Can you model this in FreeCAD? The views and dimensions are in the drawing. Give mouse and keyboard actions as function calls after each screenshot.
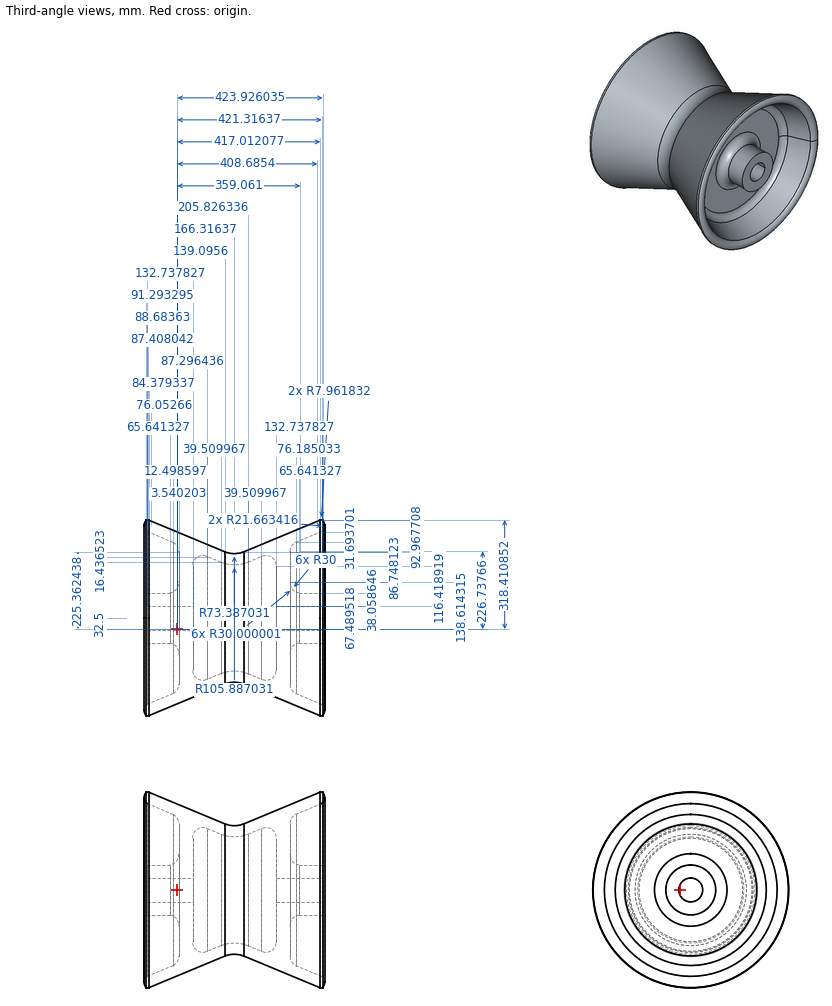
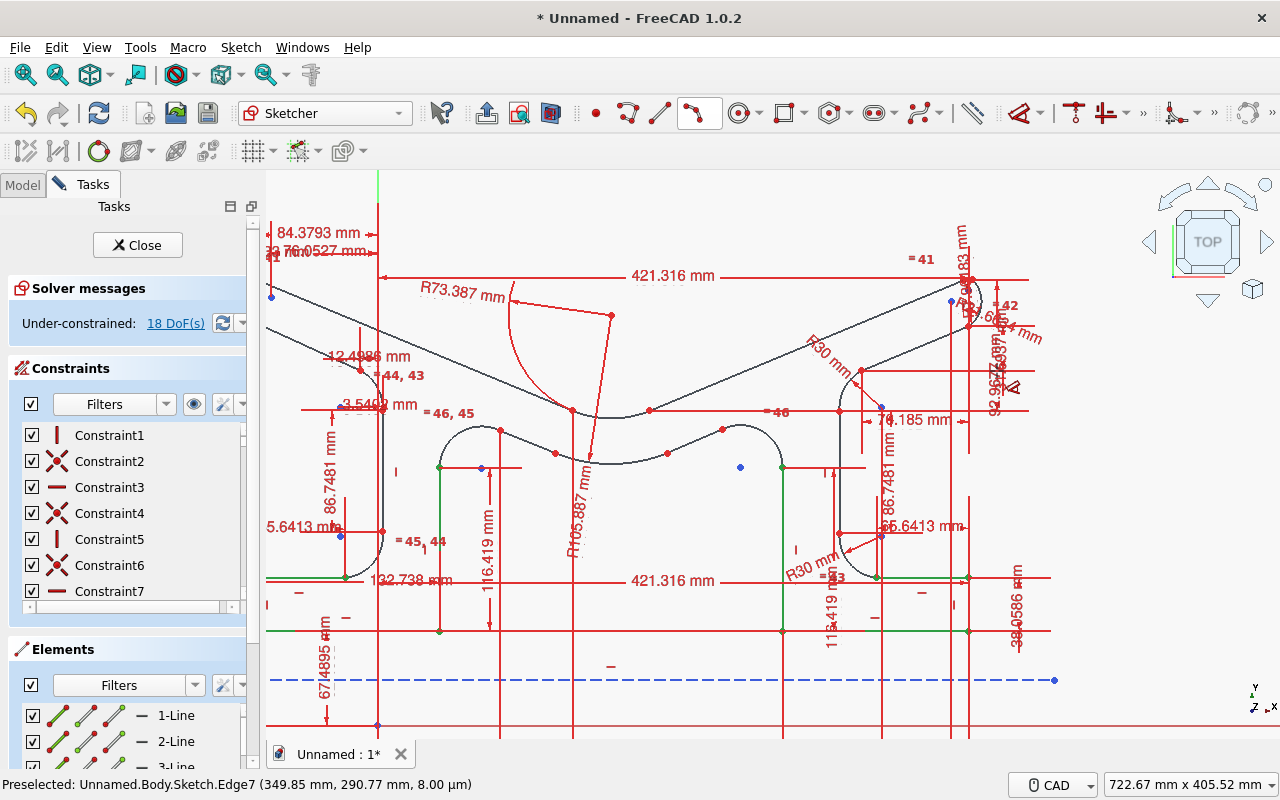
click(479, 372)
click(607, 346)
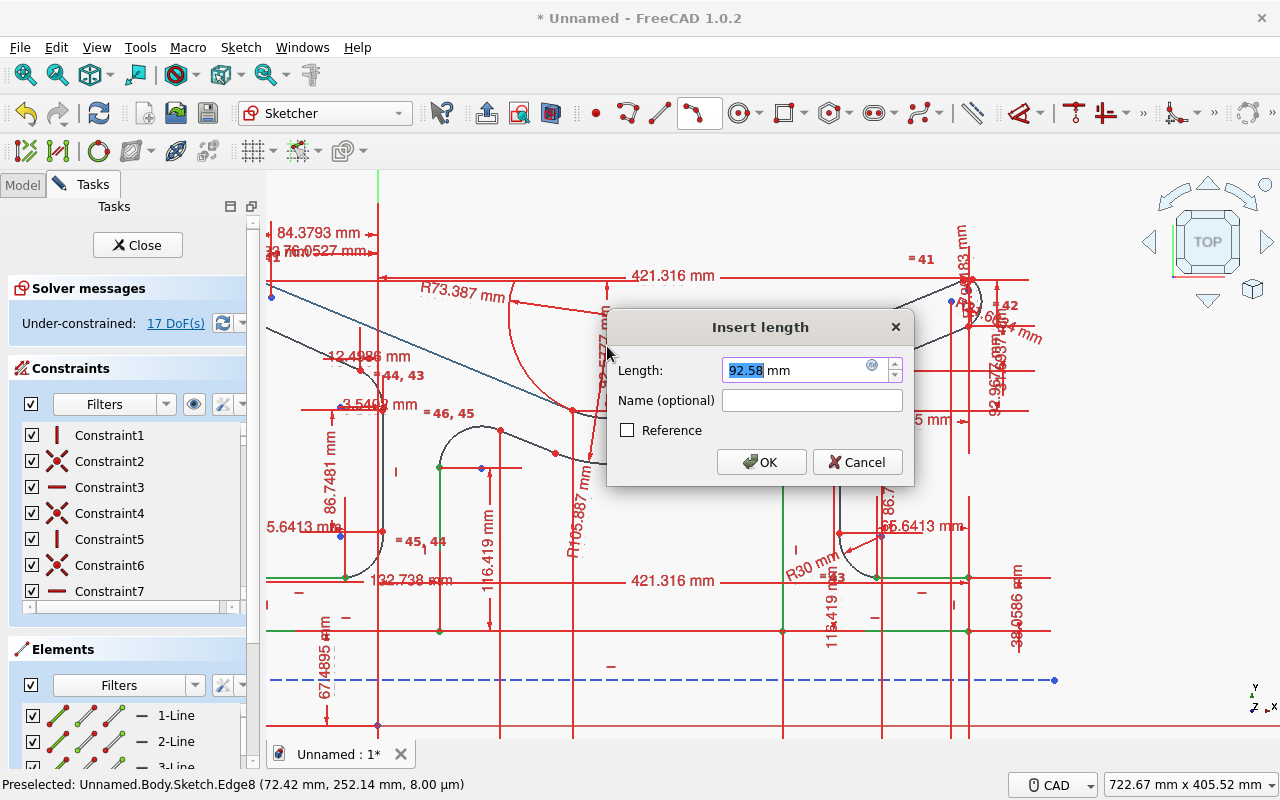
text(92.967708)
key(Return)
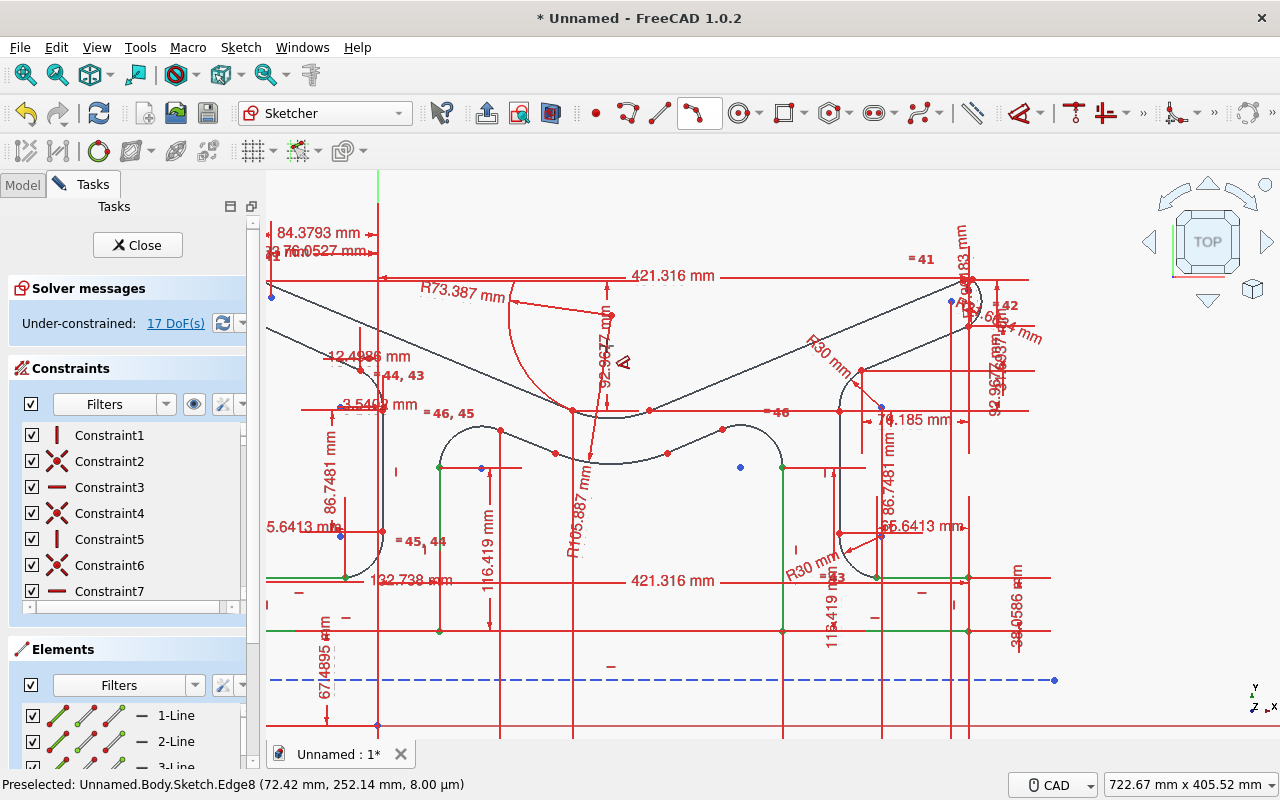
click(328, 356)
click(418, 329)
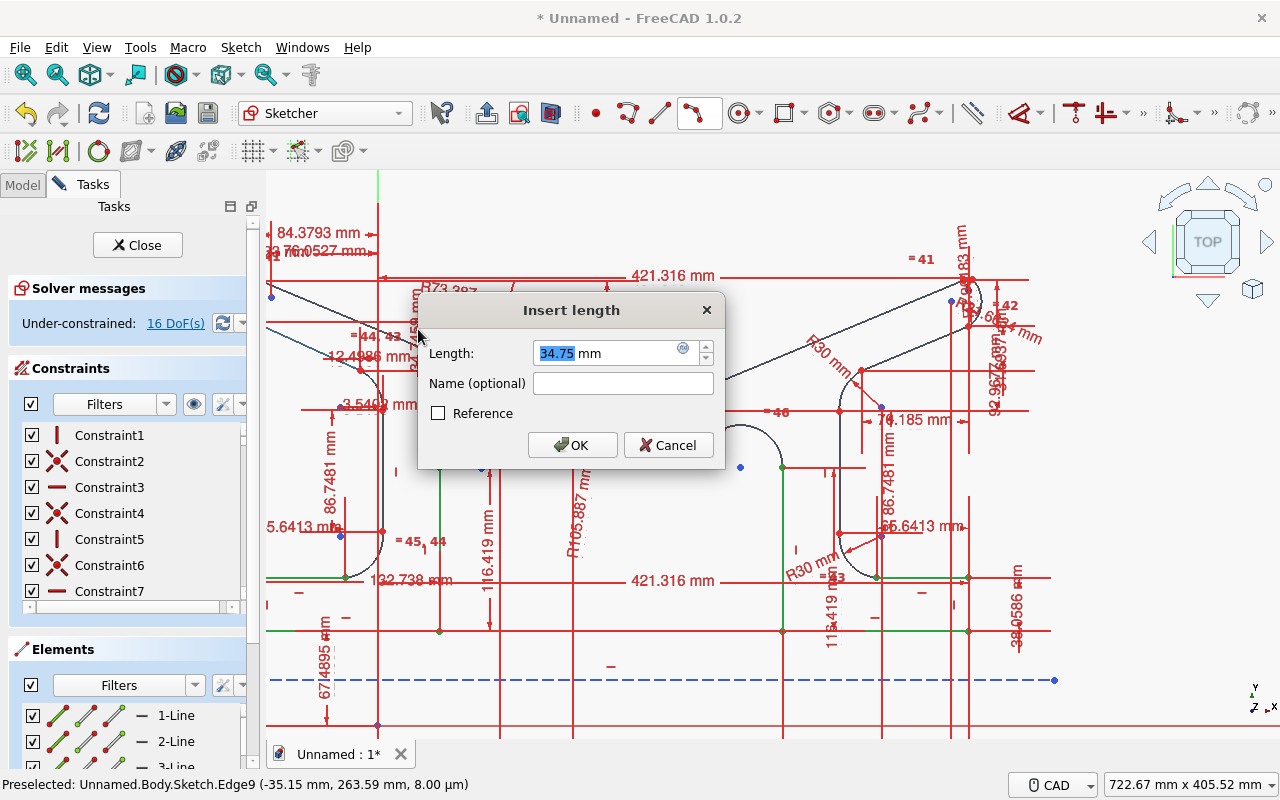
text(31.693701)
key(Return)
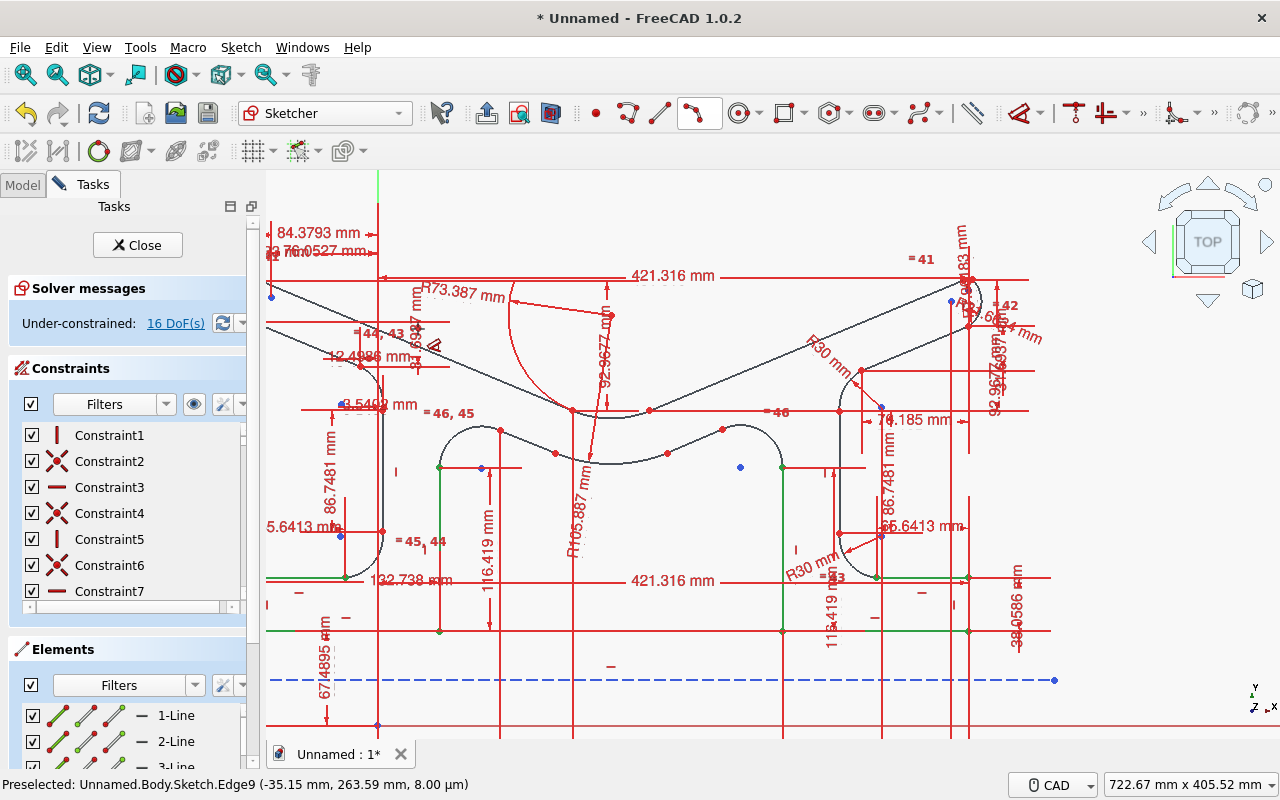
click(517, 437)
click(528, 487)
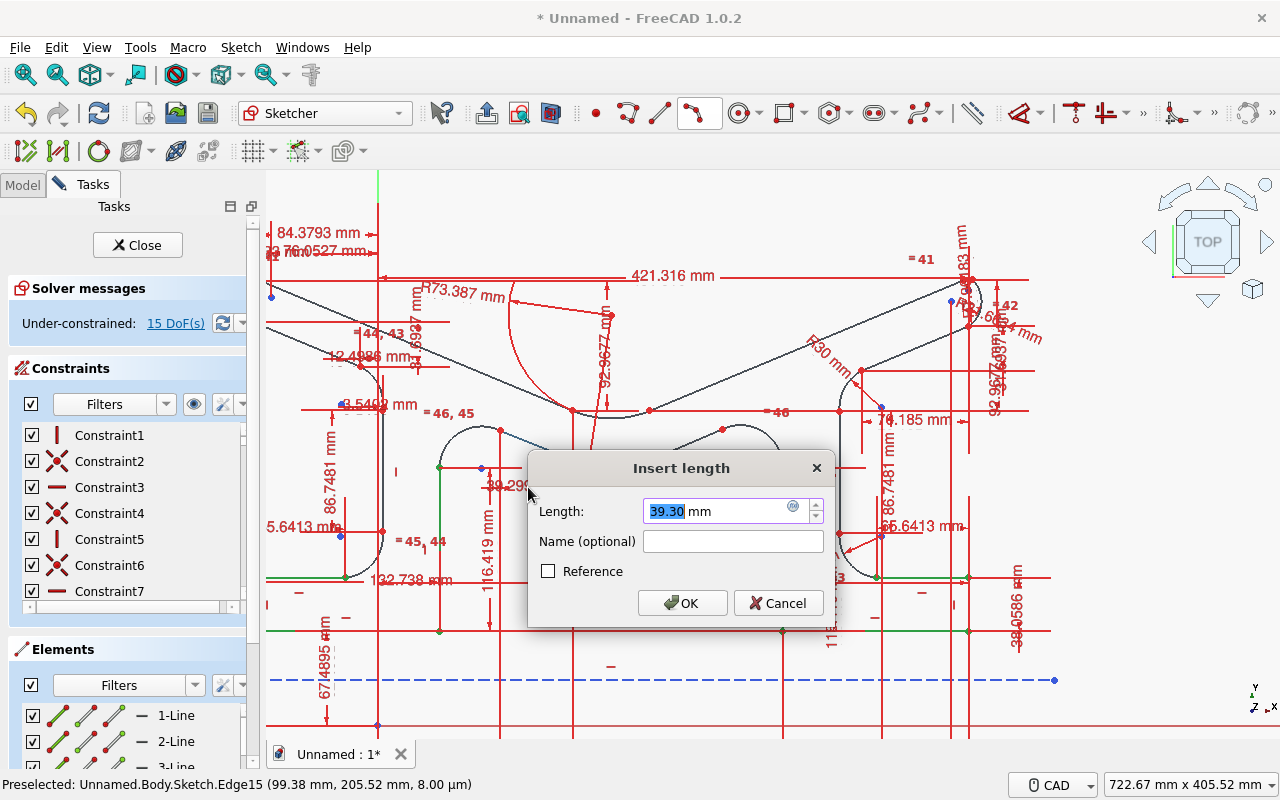
text(39.509967)
key(Return)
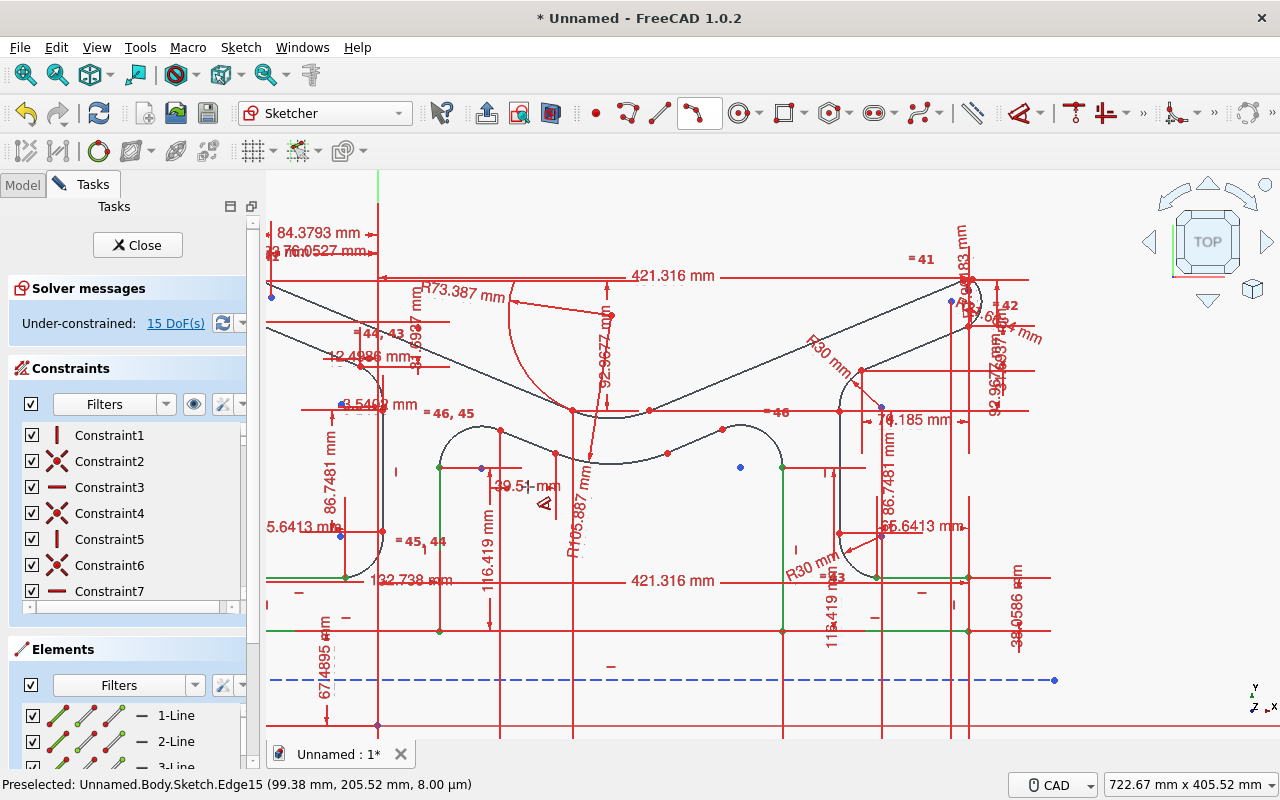
scroll(517, 437, up, 3)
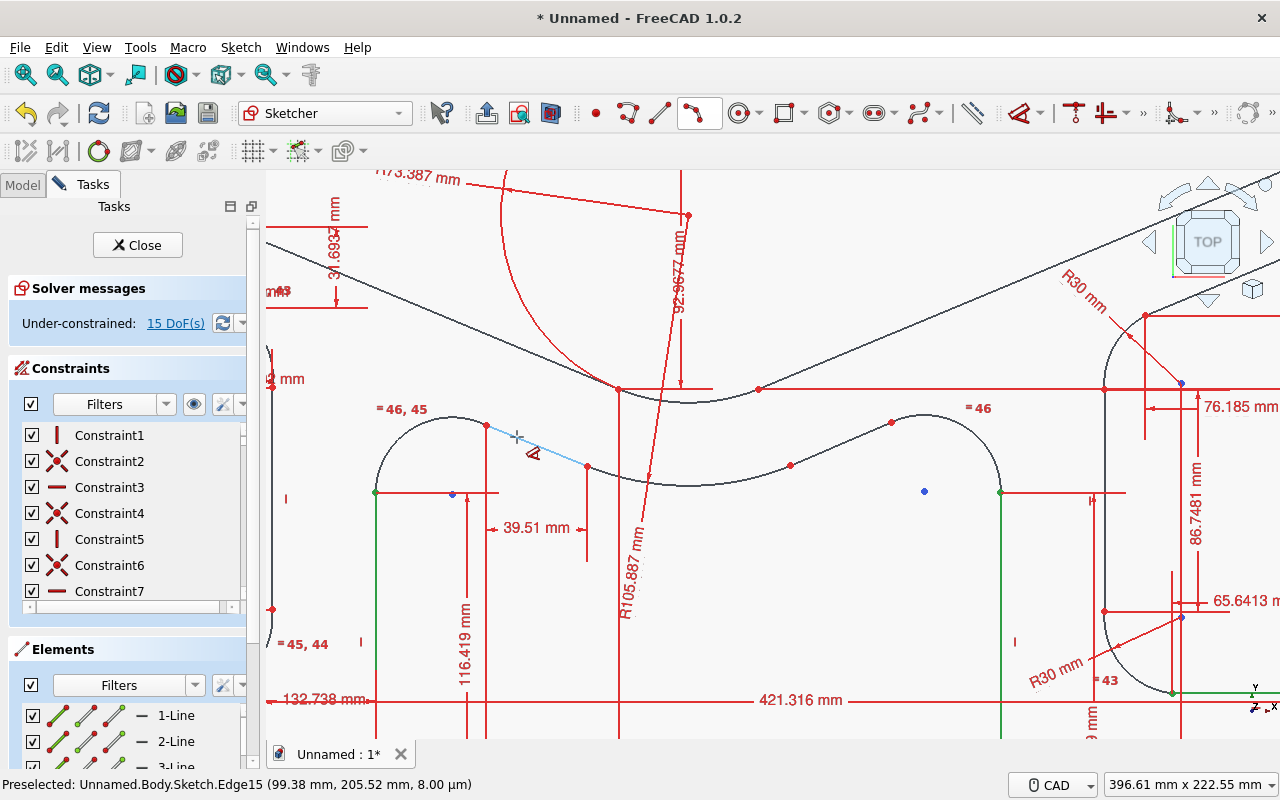
click(516, 438)
click(452, 446)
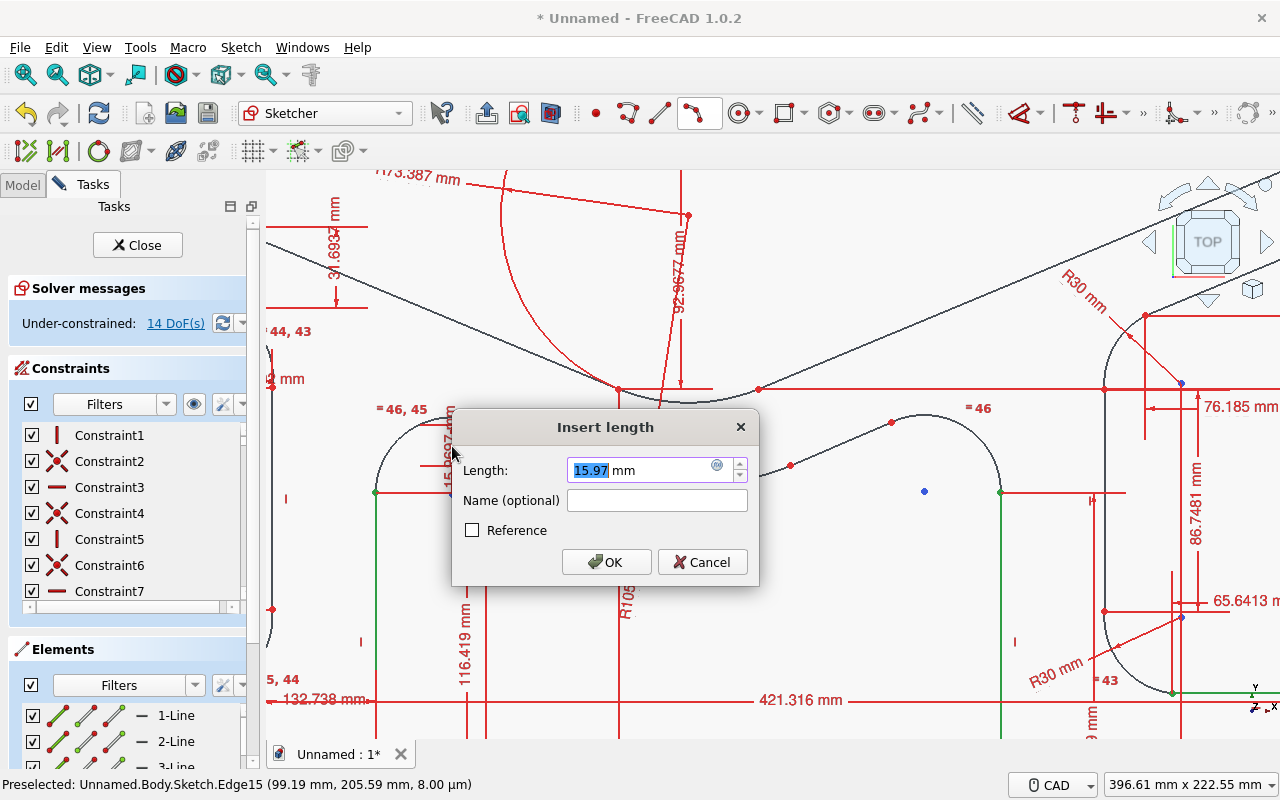
text(16.436523)
key(Return)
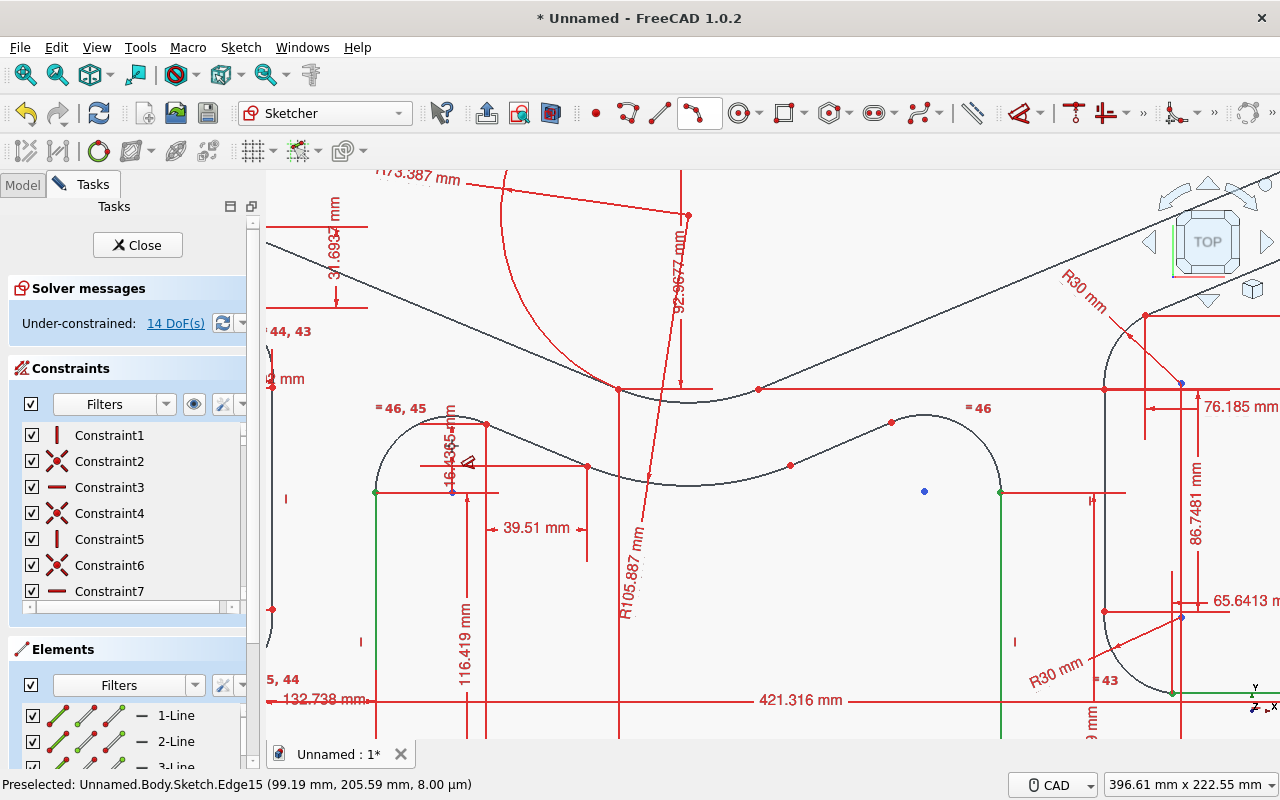
click(821, 453)
click(841, 389)